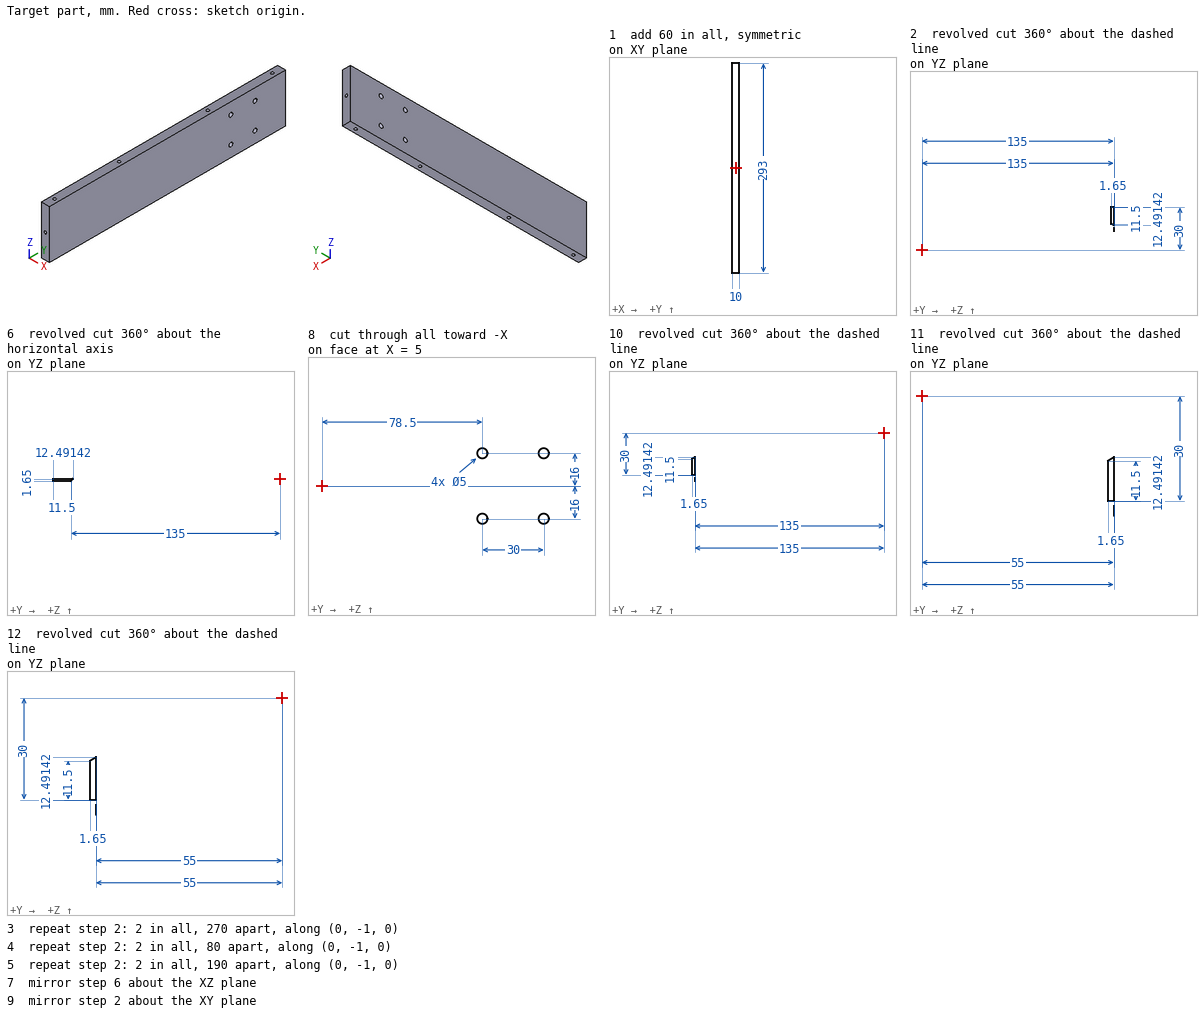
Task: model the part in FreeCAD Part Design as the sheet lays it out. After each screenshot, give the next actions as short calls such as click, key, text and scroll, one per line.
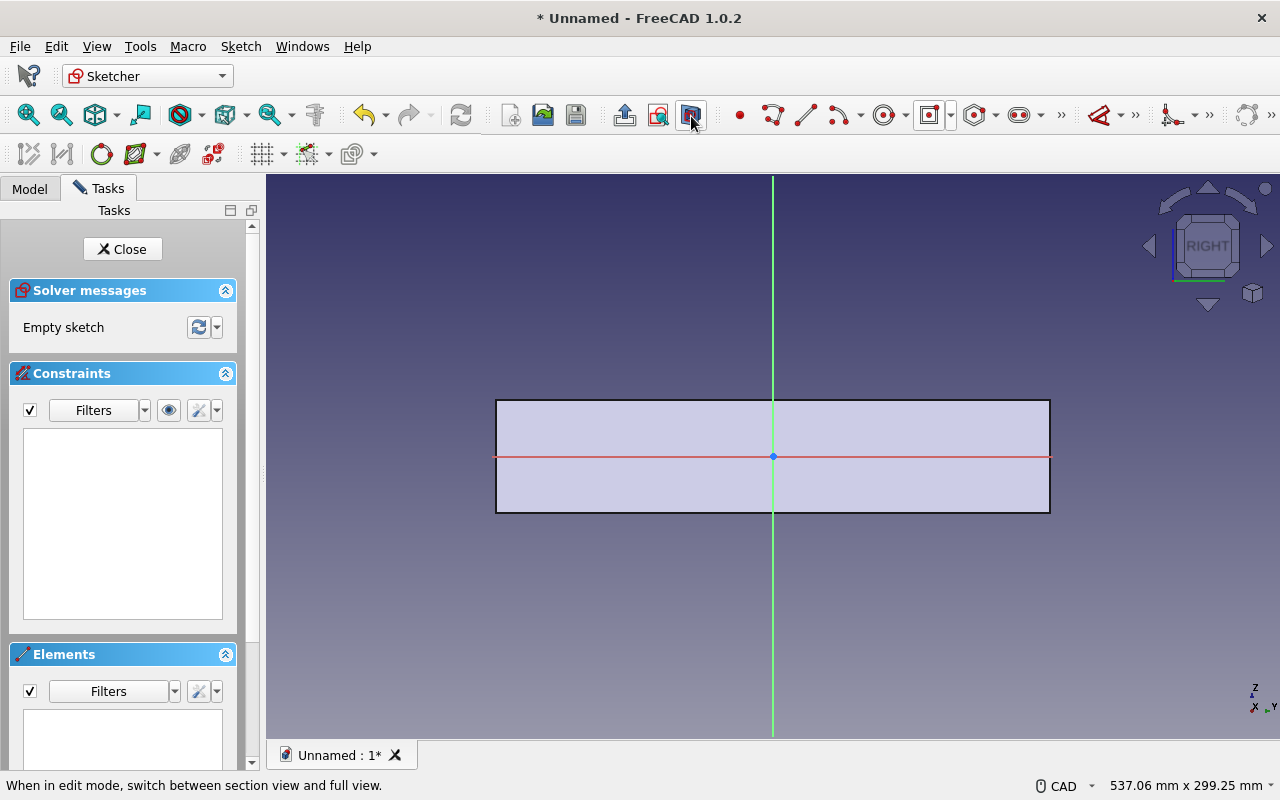
scroll(1058, 412, up, 12)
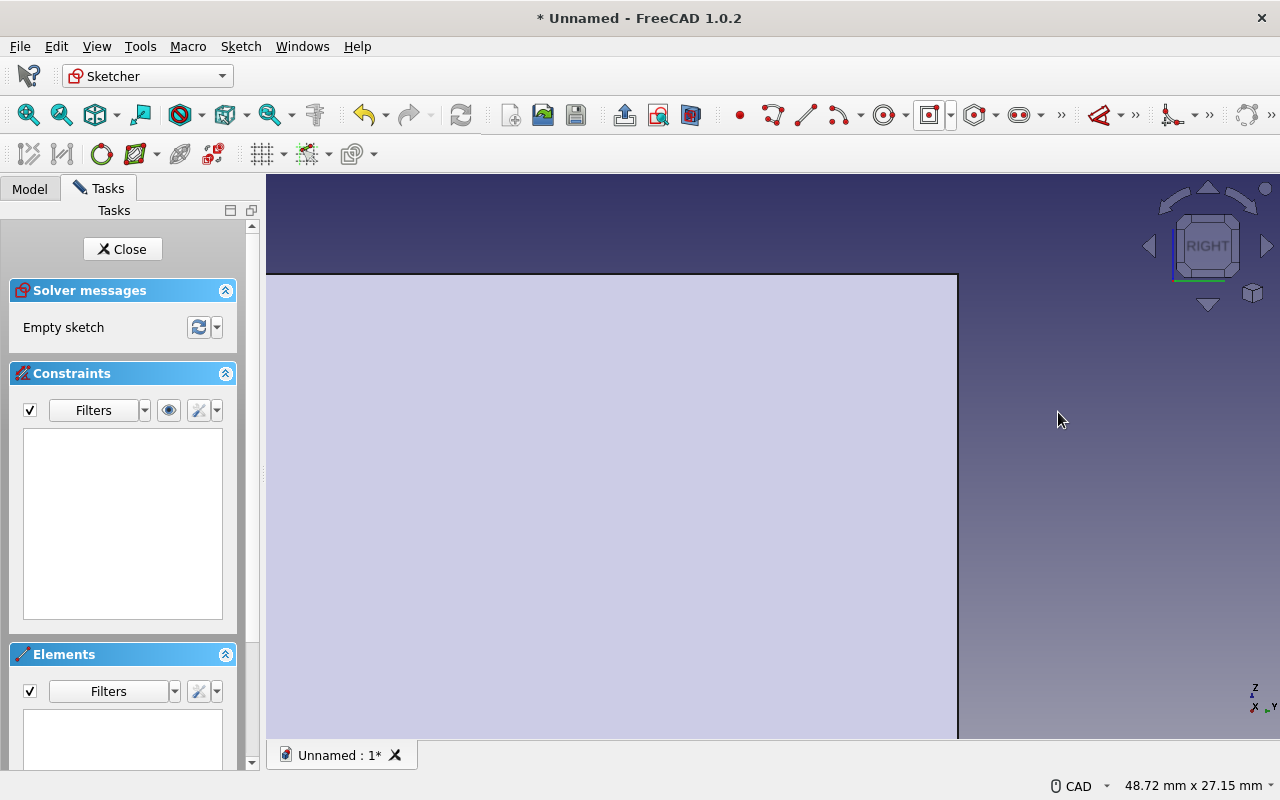
click(773, 116)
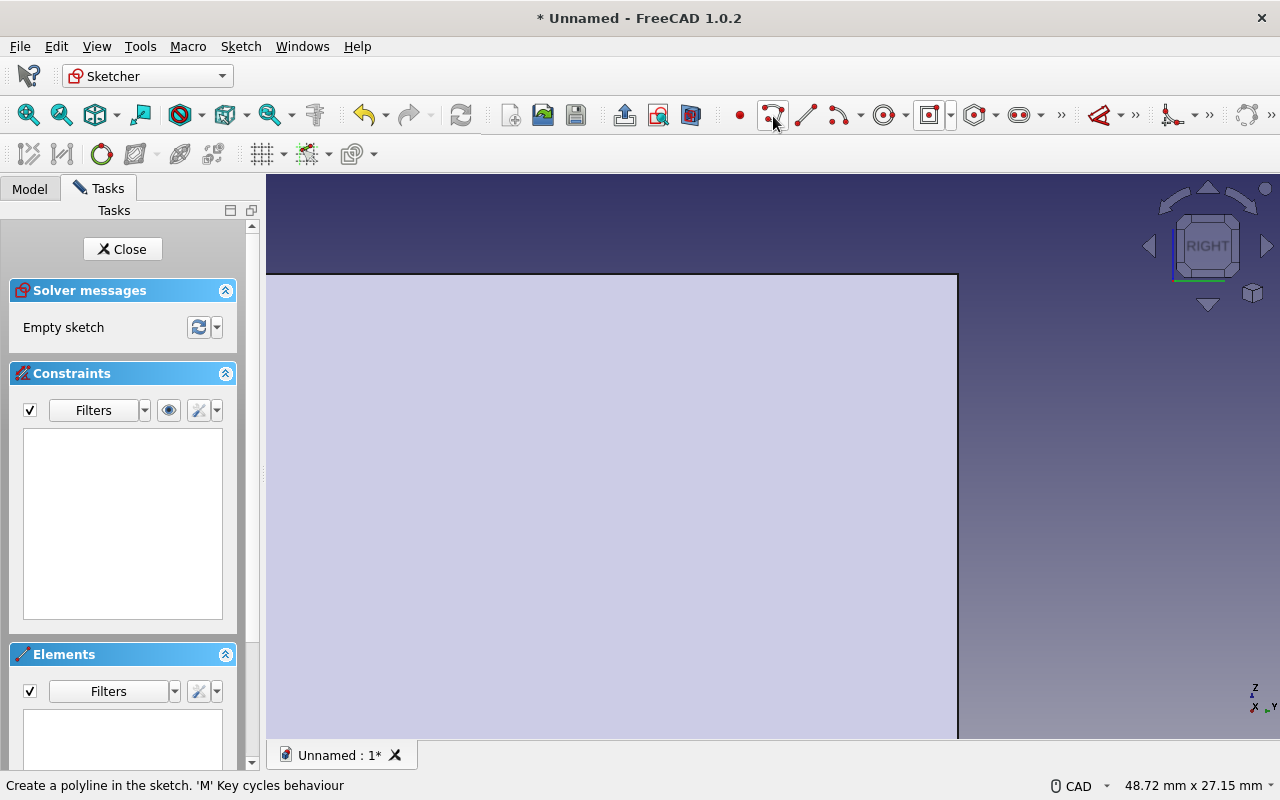
click(684, 513)
click(718, 534)
click(718, 274)
click(684, 274)
click(684, 514)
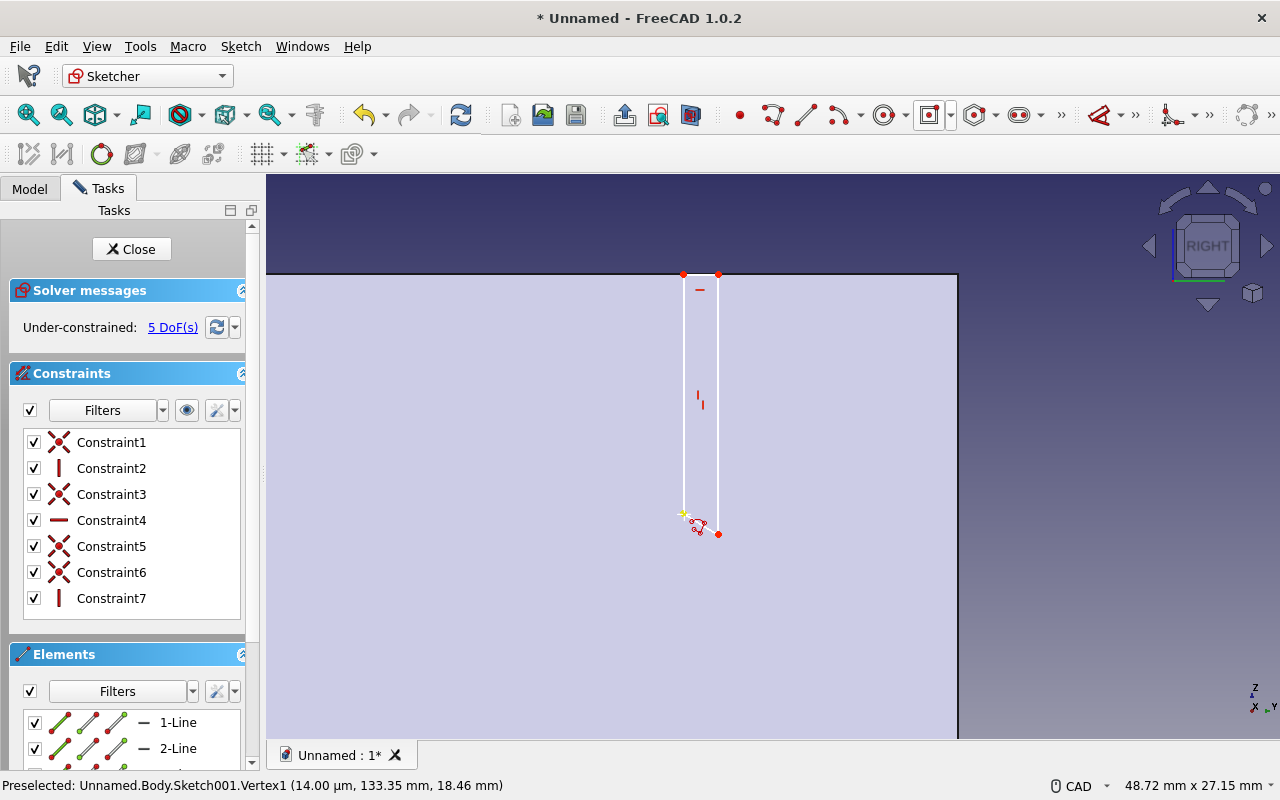
click(806, 116)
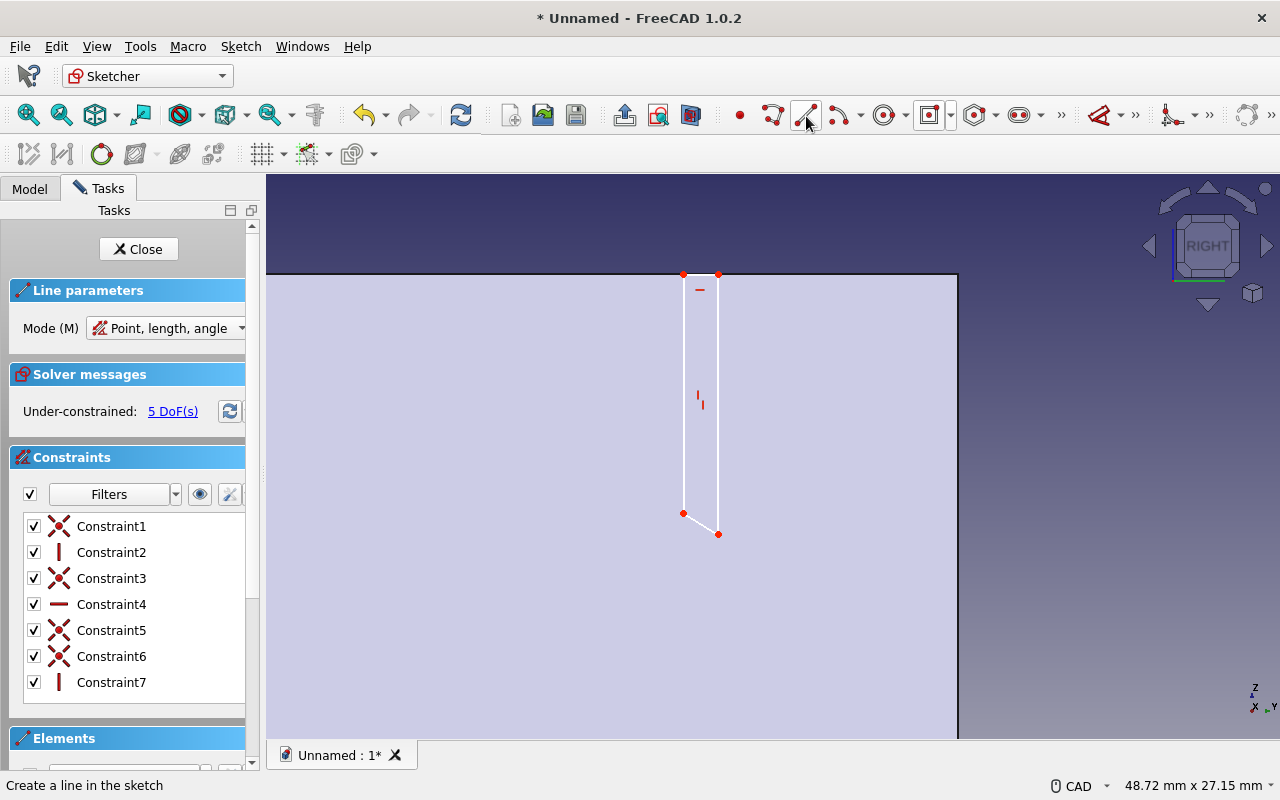
click(718, 560)
click(718, 638)
key(Escape)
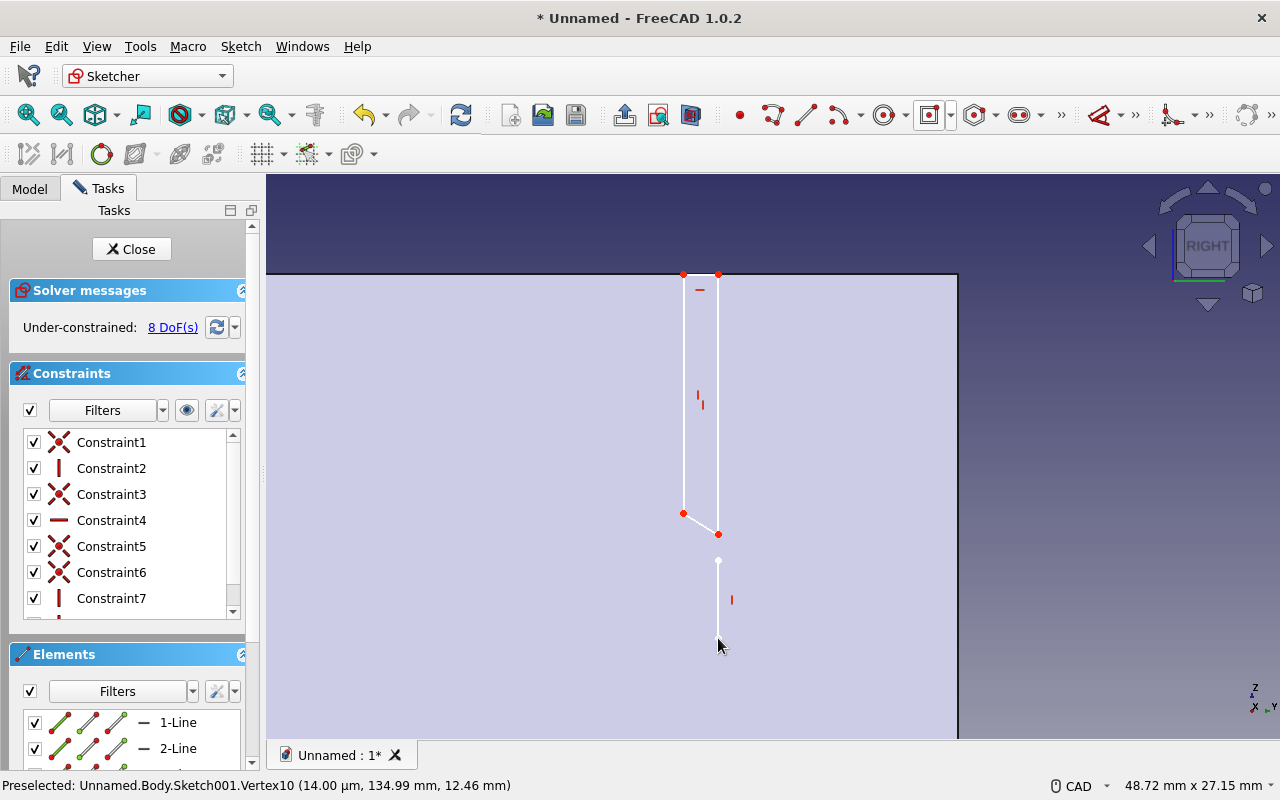
click(718, 584)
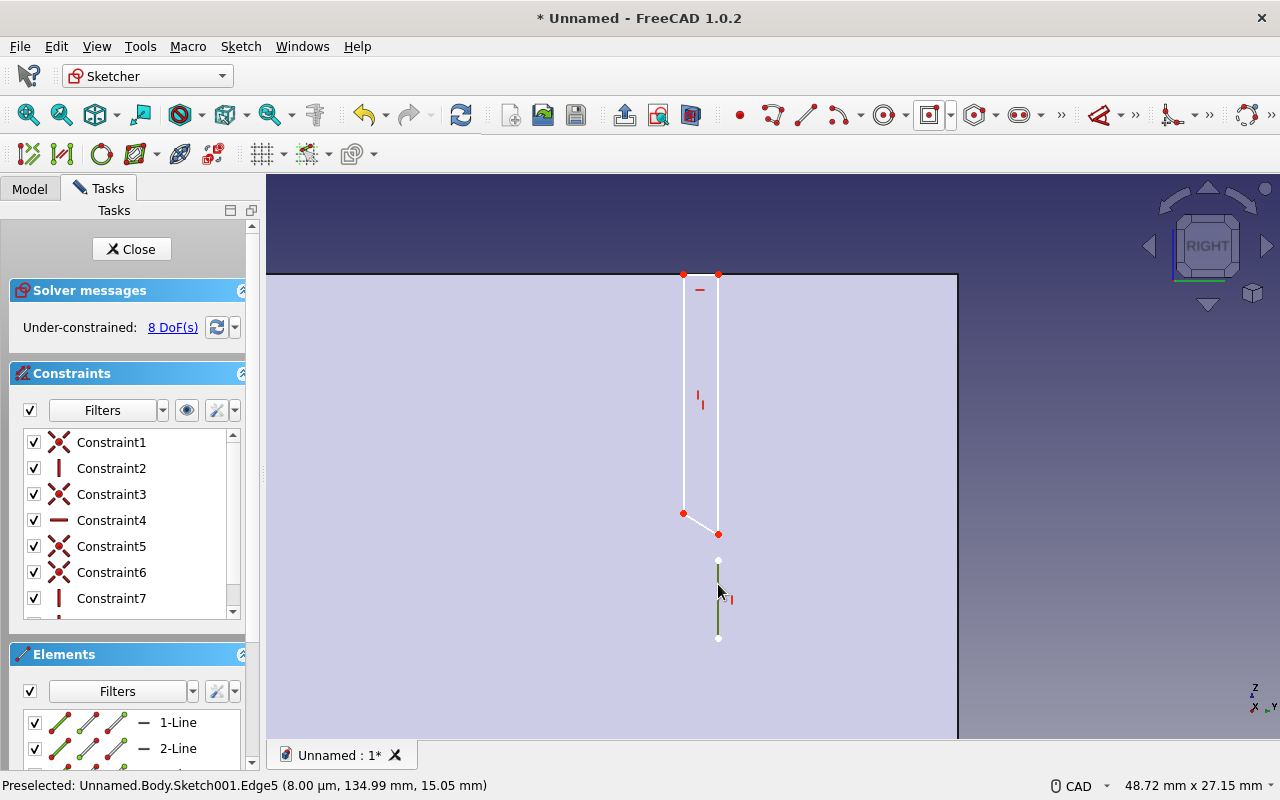
key(g)
key(n)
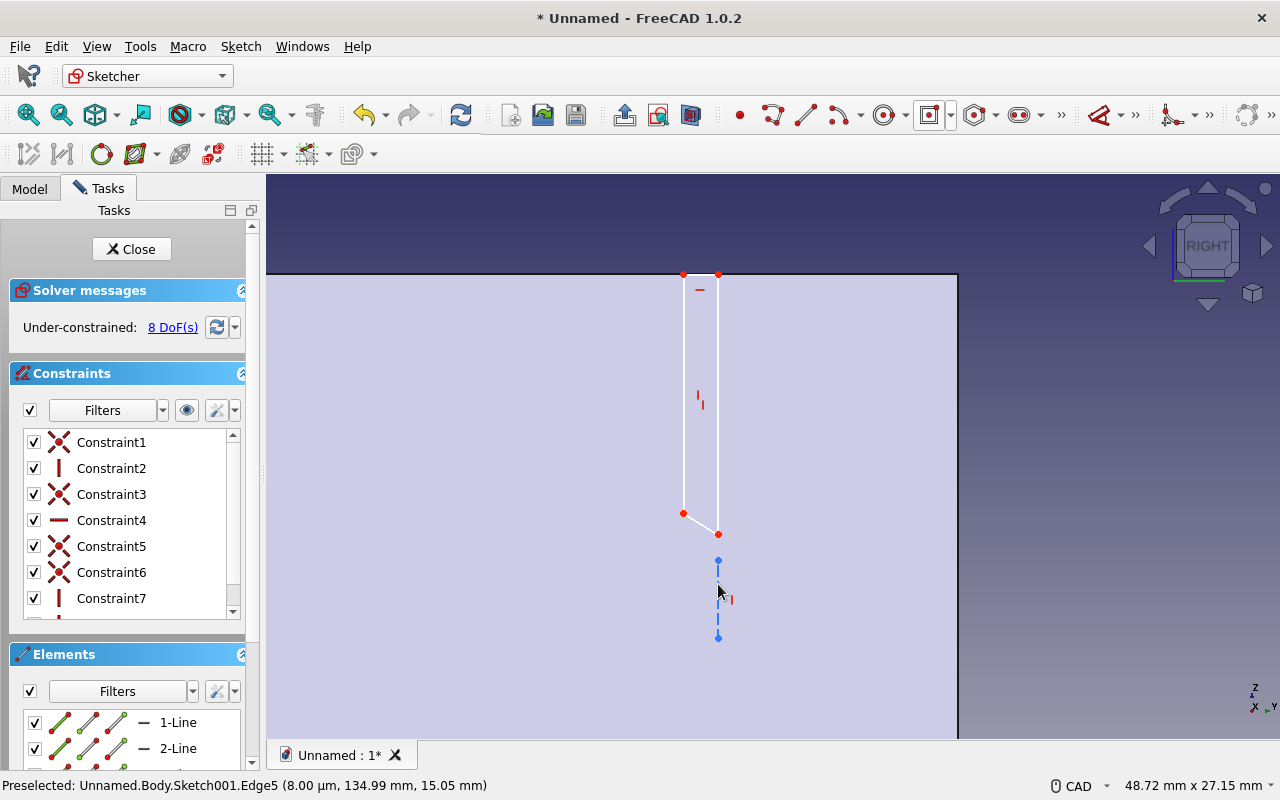
click(718, 275)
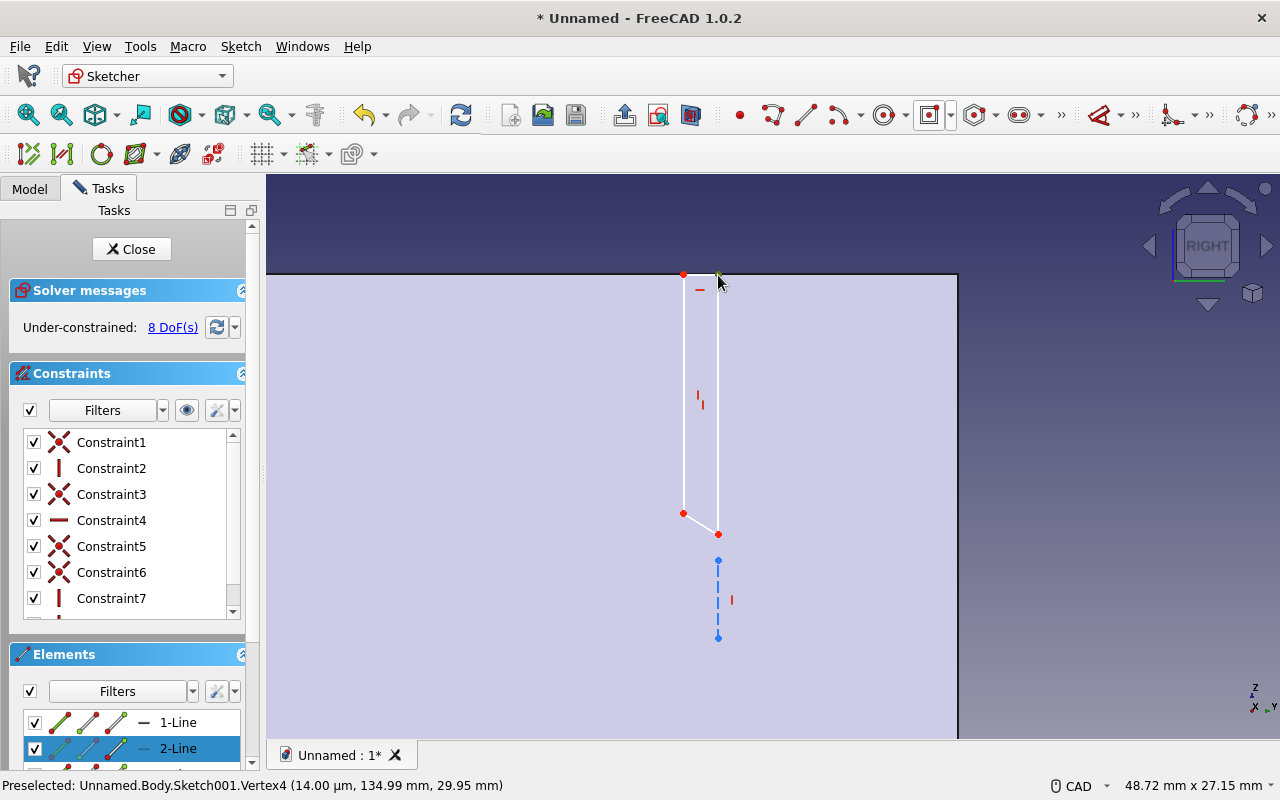
click(1120, 116)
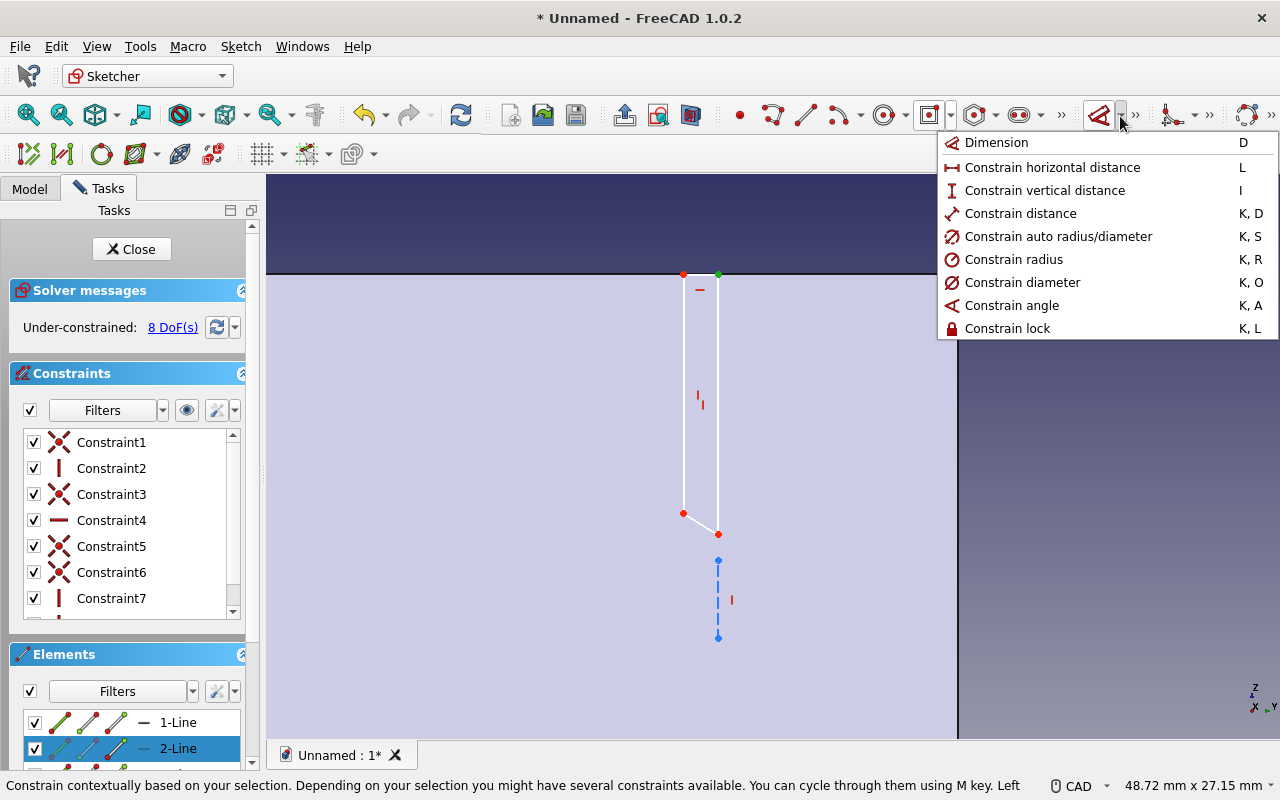
click(1108, 190)